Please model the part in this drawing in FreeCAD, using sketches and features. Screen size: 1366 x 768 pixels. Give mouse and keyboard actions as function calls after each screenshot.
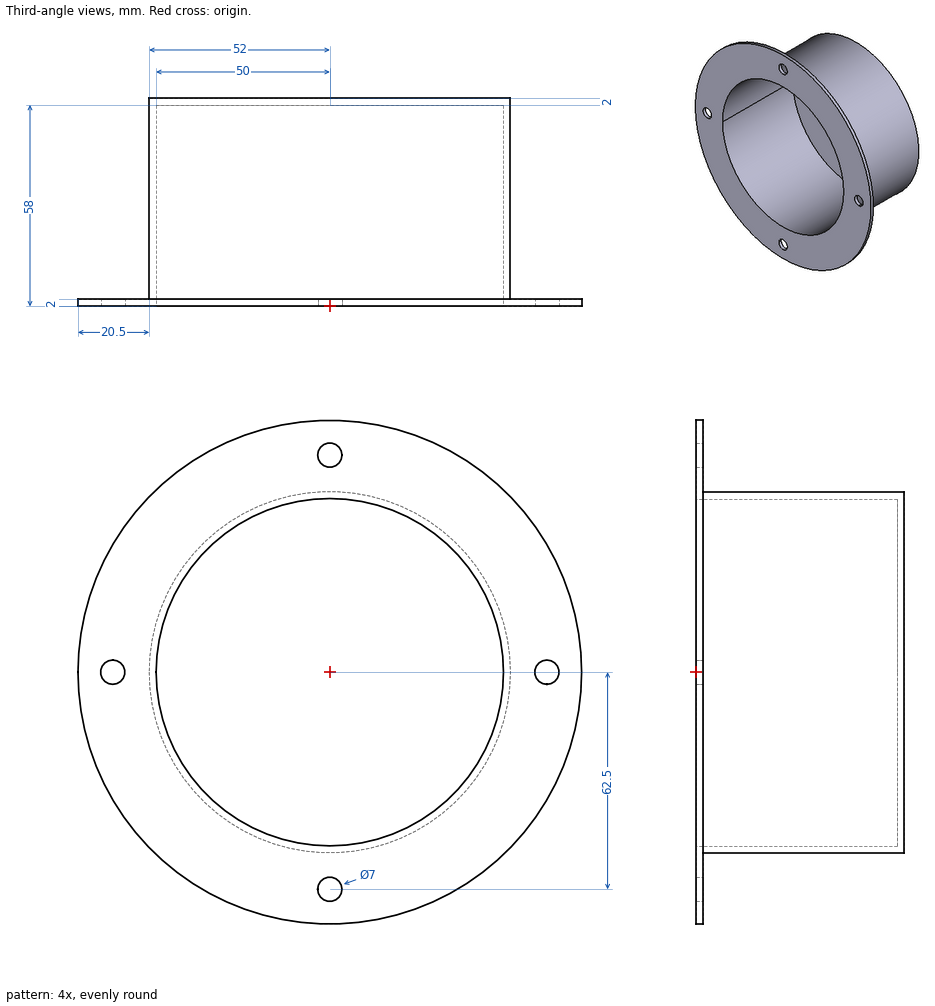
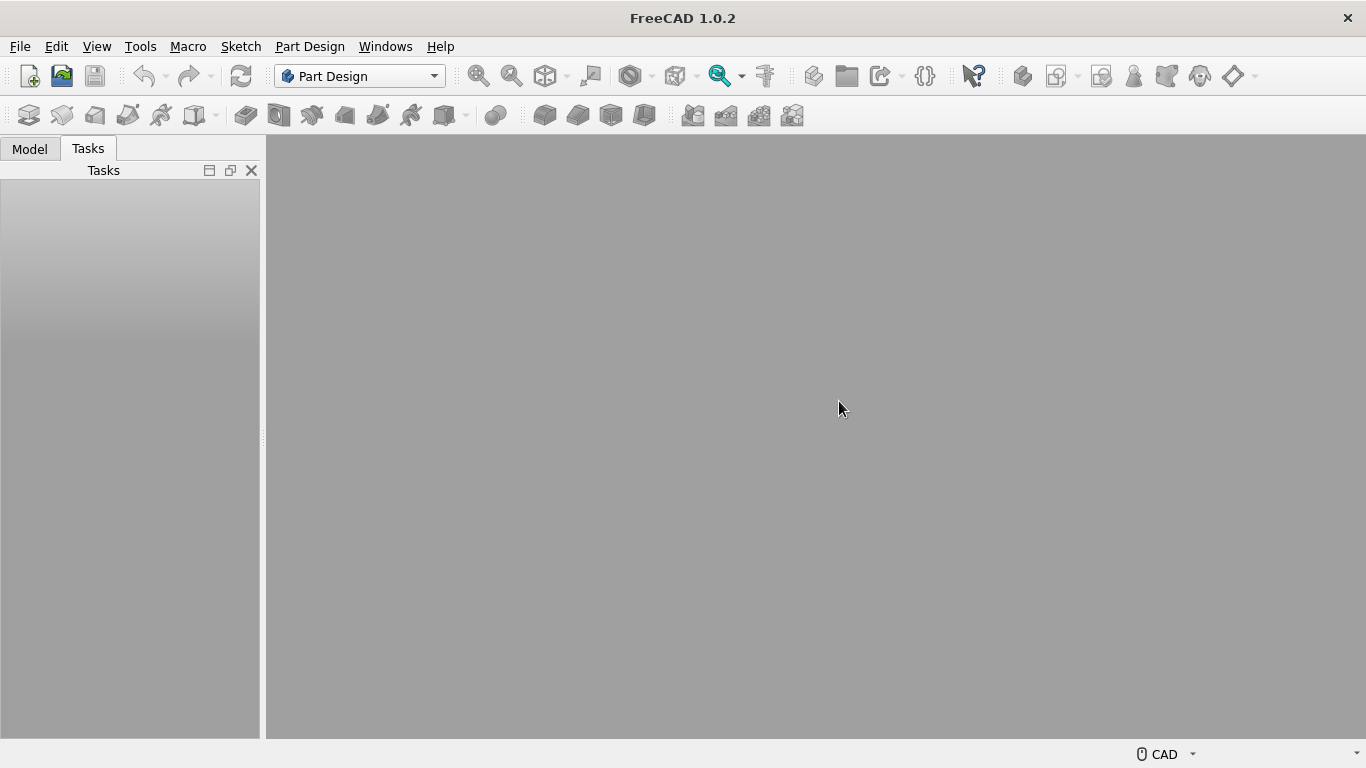
click(29, 76)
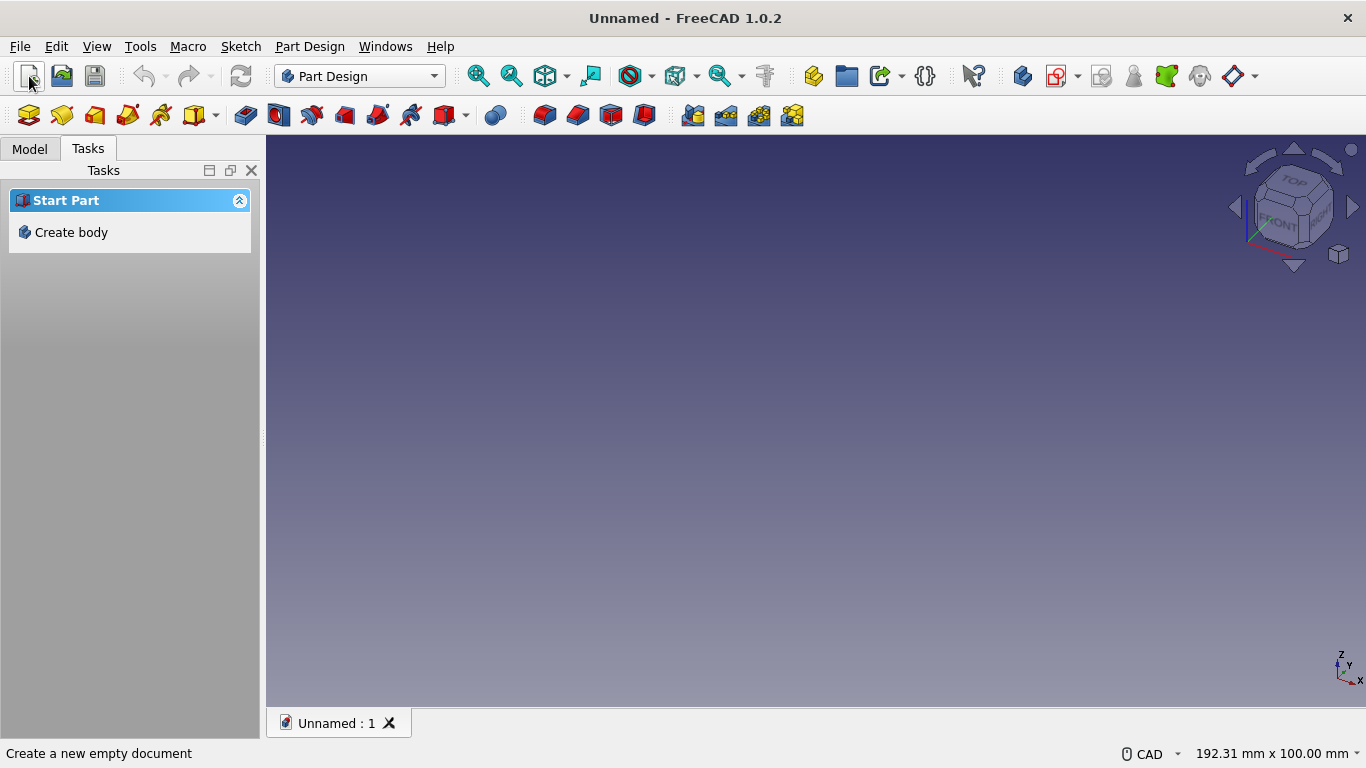
click(1056, 76)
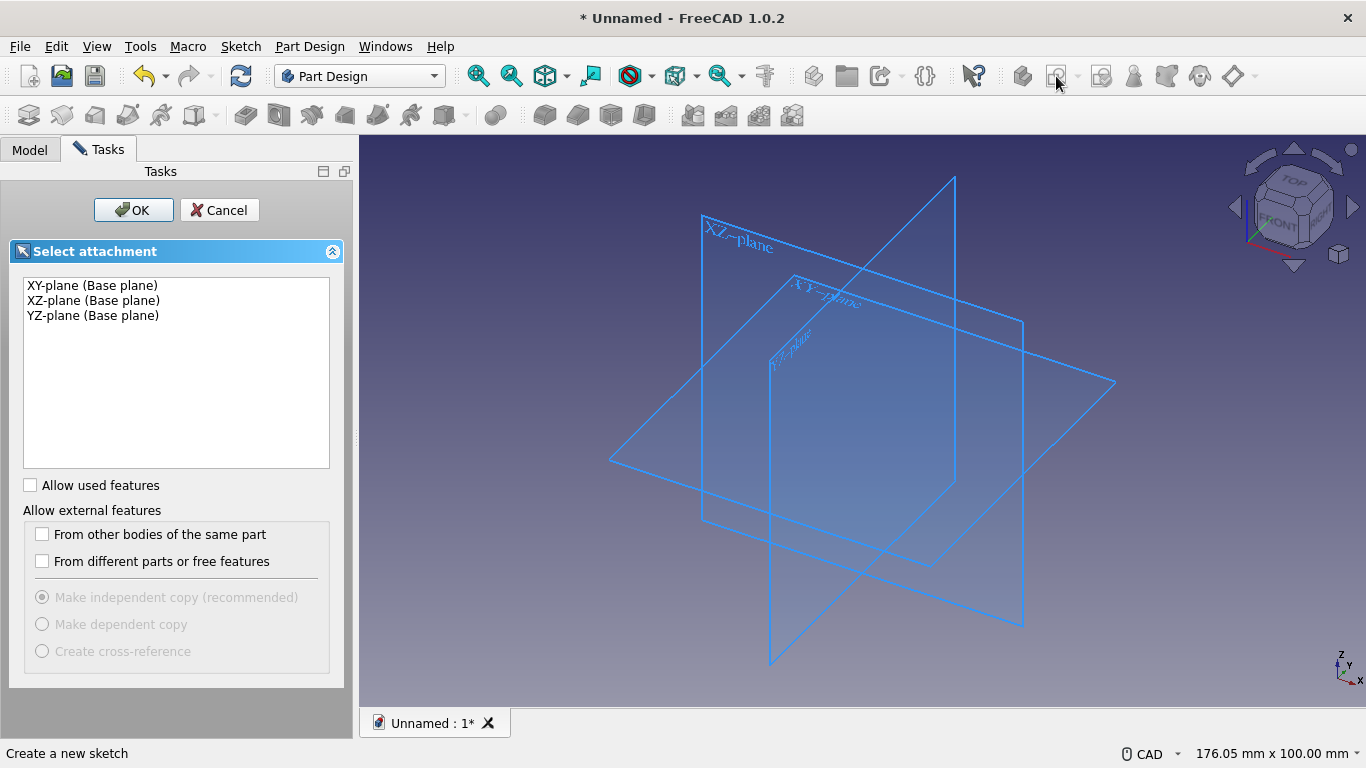
click(84, 286)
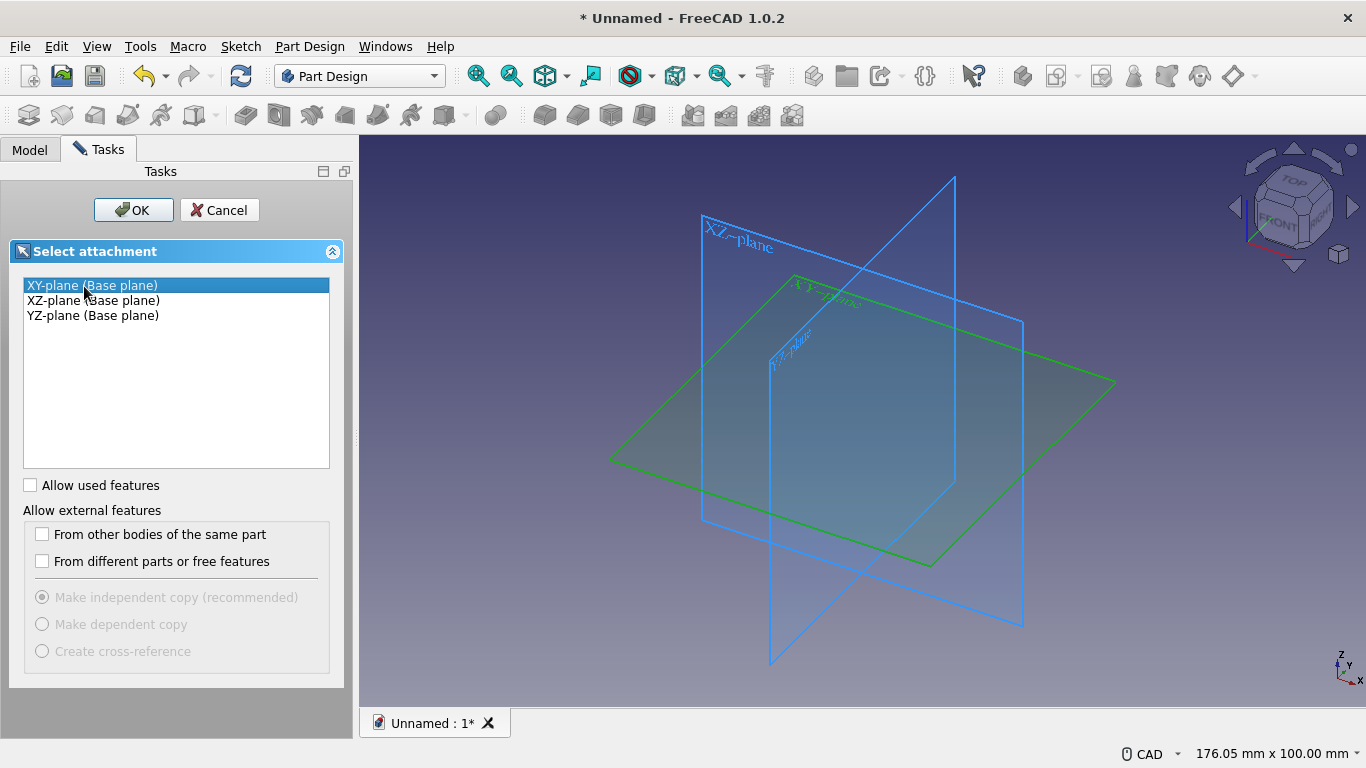
click(134, 210)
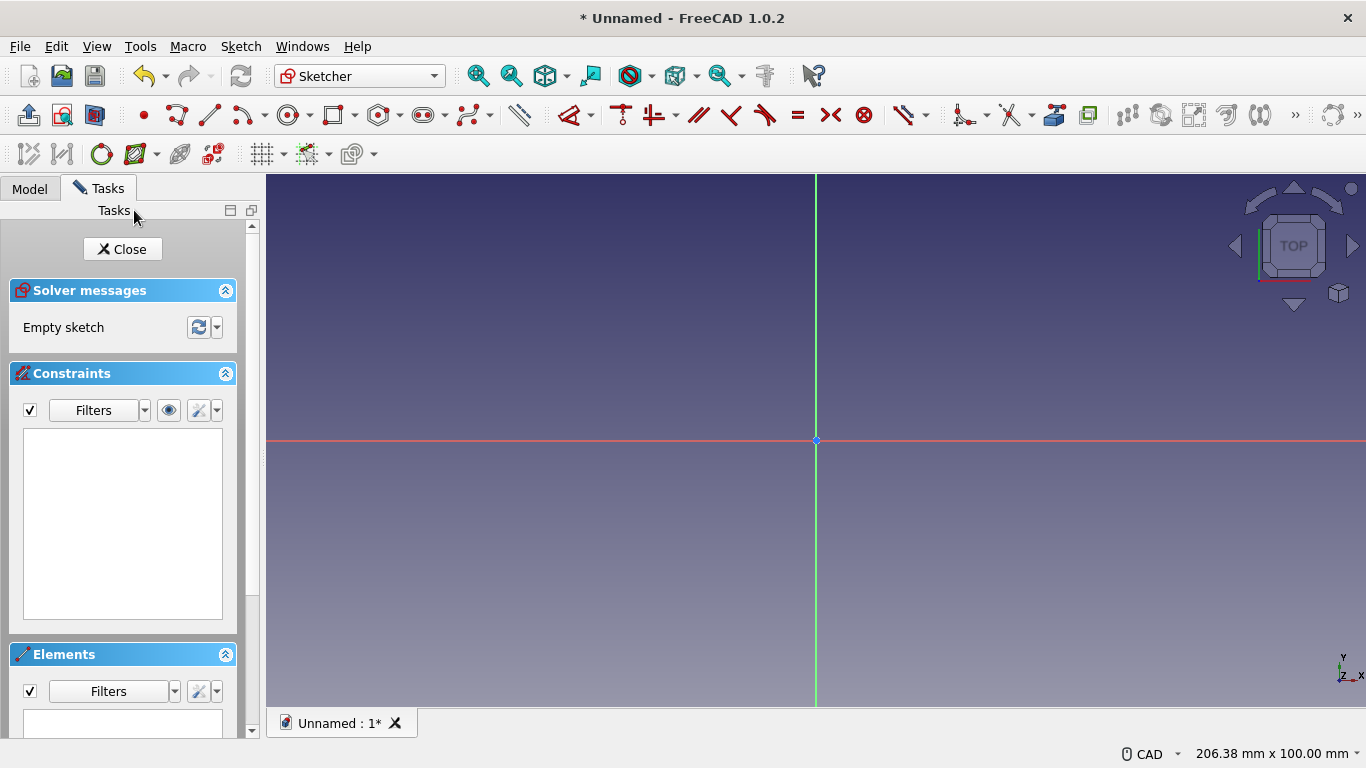
scroll(1001, 679, down, 2)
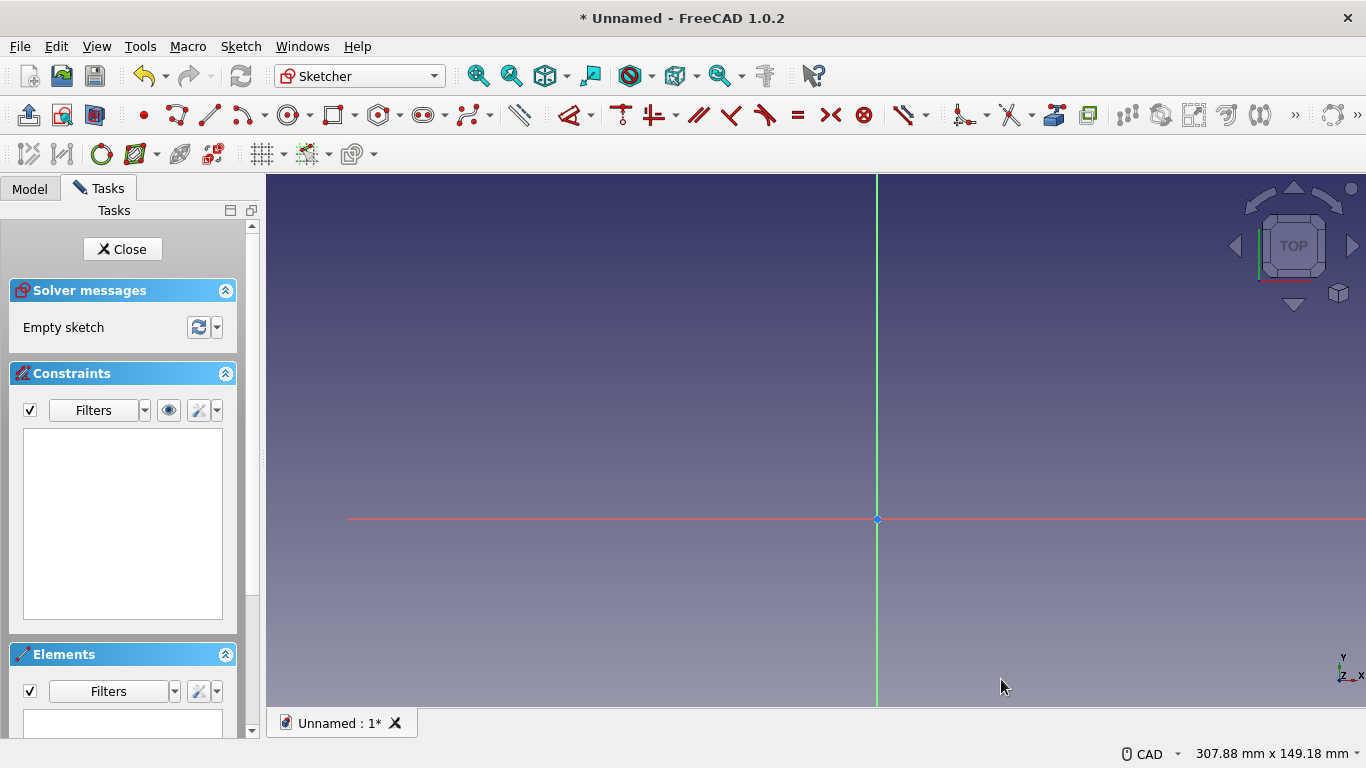
scroll(748, 355, up, 2)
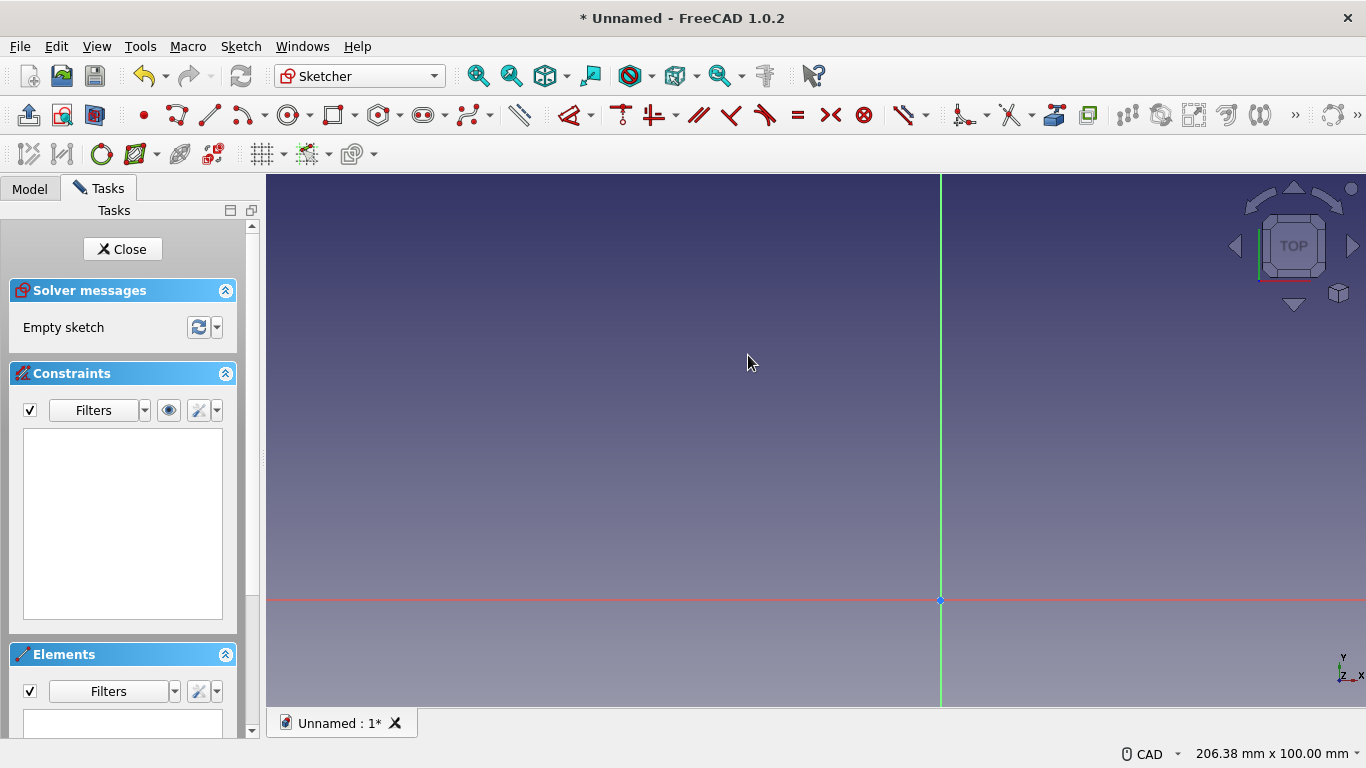
key(g)
key(m)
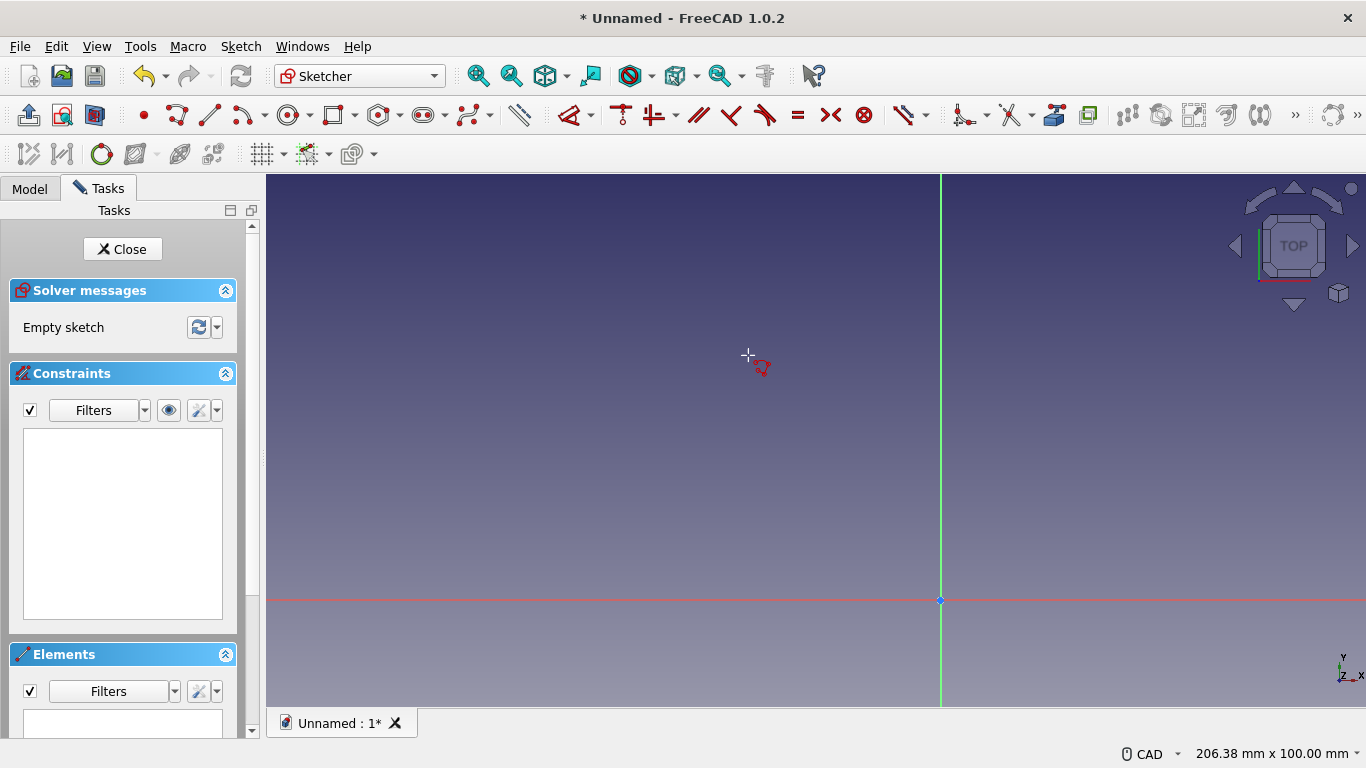
click(674, 600)
click(674, 291)
click(941, 291)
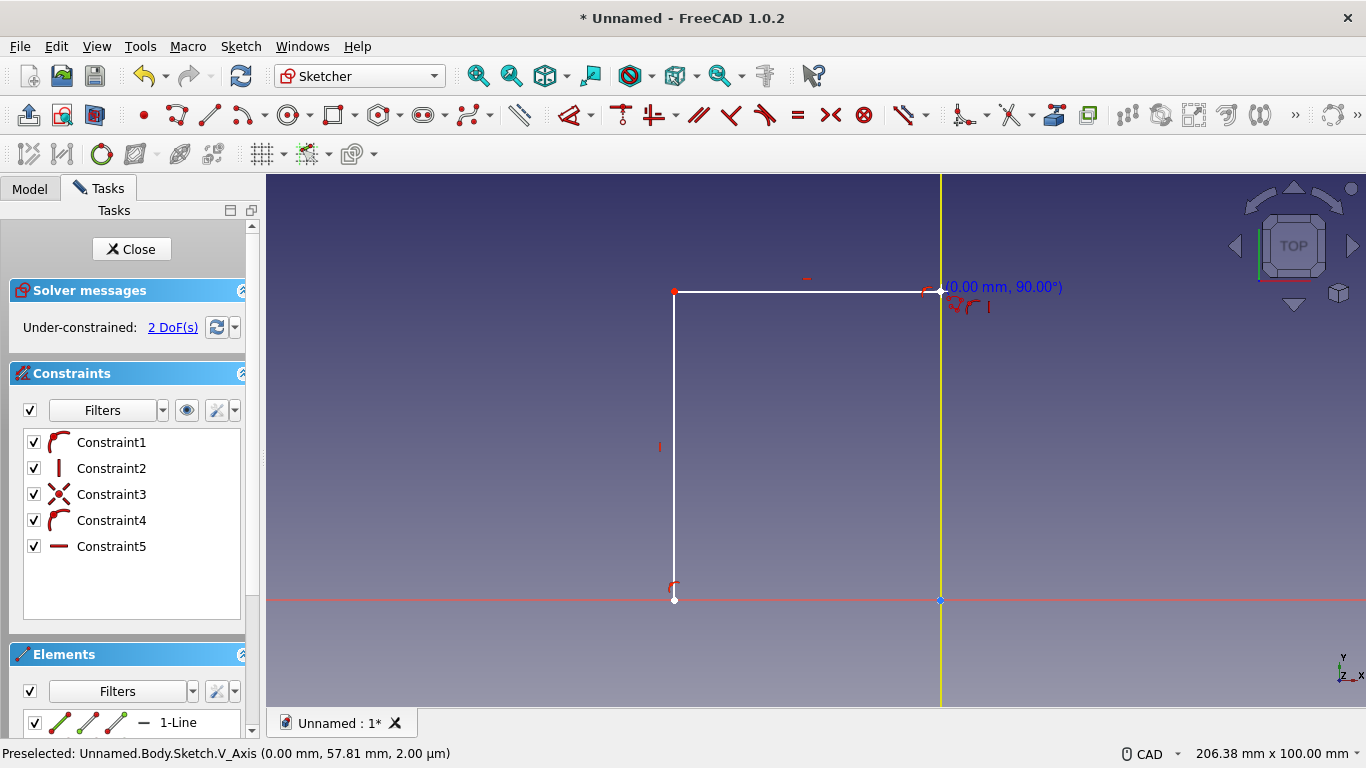
scroll(941, 280, up, 2)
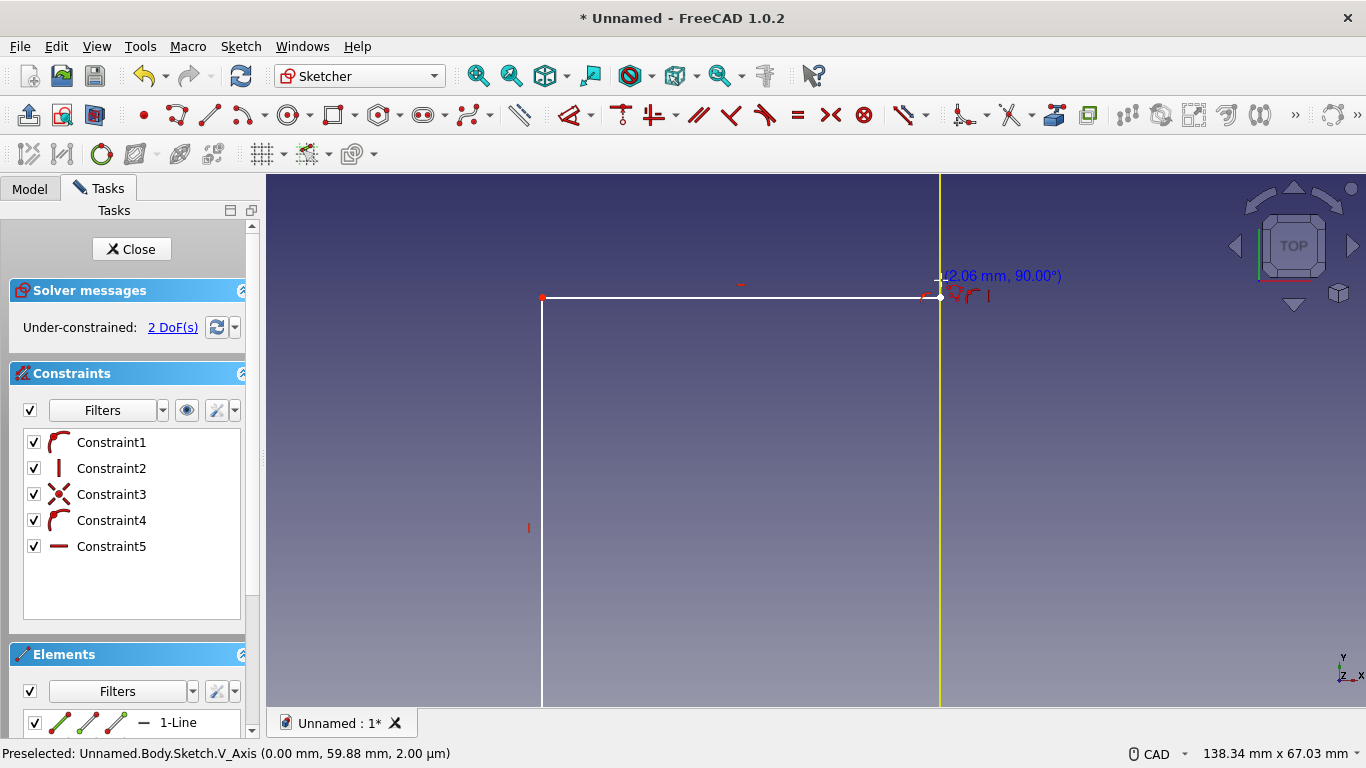
click(931, 280)
click(527, 280)